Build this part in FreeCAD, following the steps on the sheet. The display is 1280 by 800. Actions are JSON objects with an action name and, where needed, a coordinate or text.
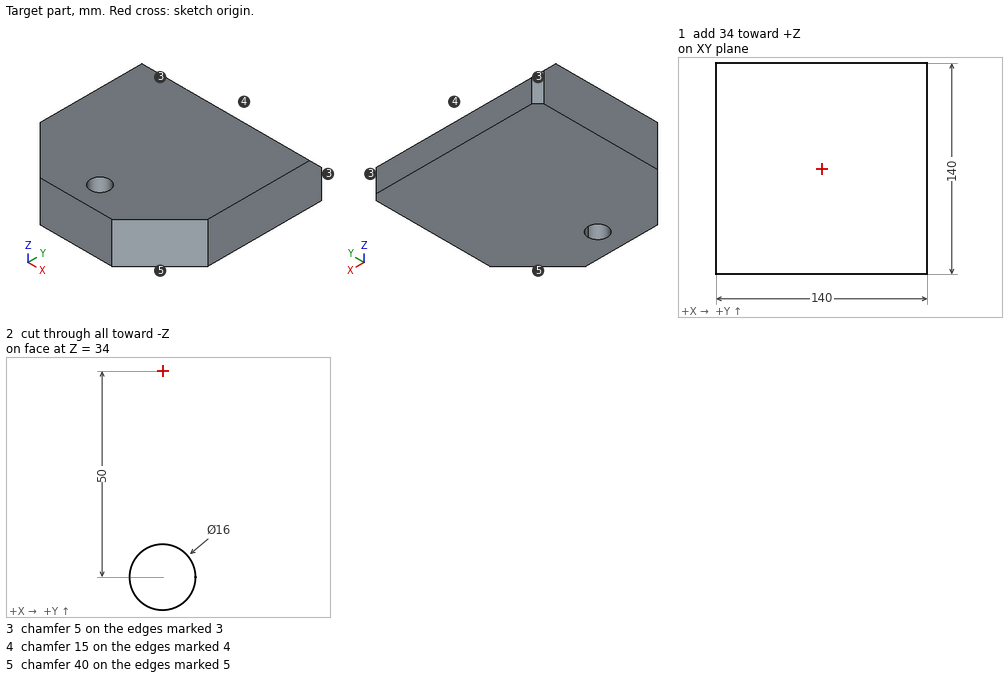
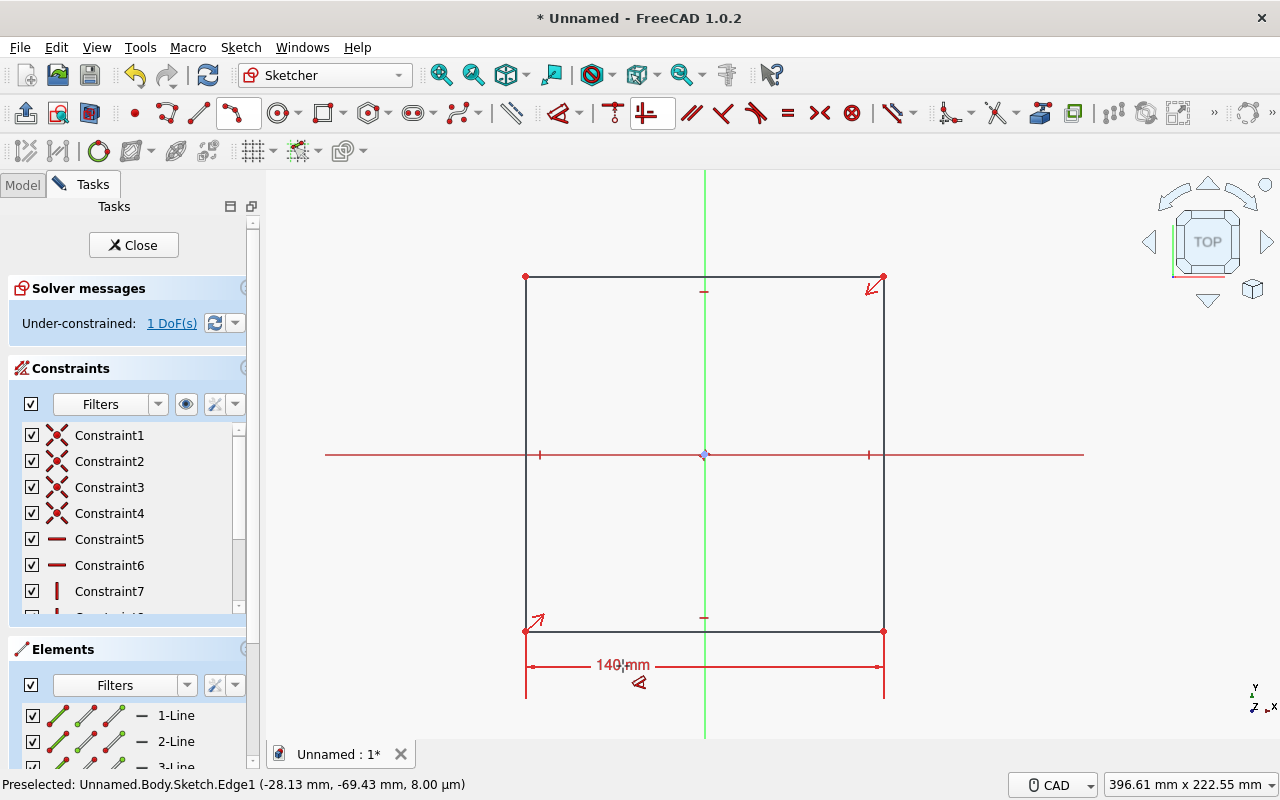
{"action": "left_click", "coordinate": [884, 526]}
{"action": "left_click", "coordinate": [918, 373]}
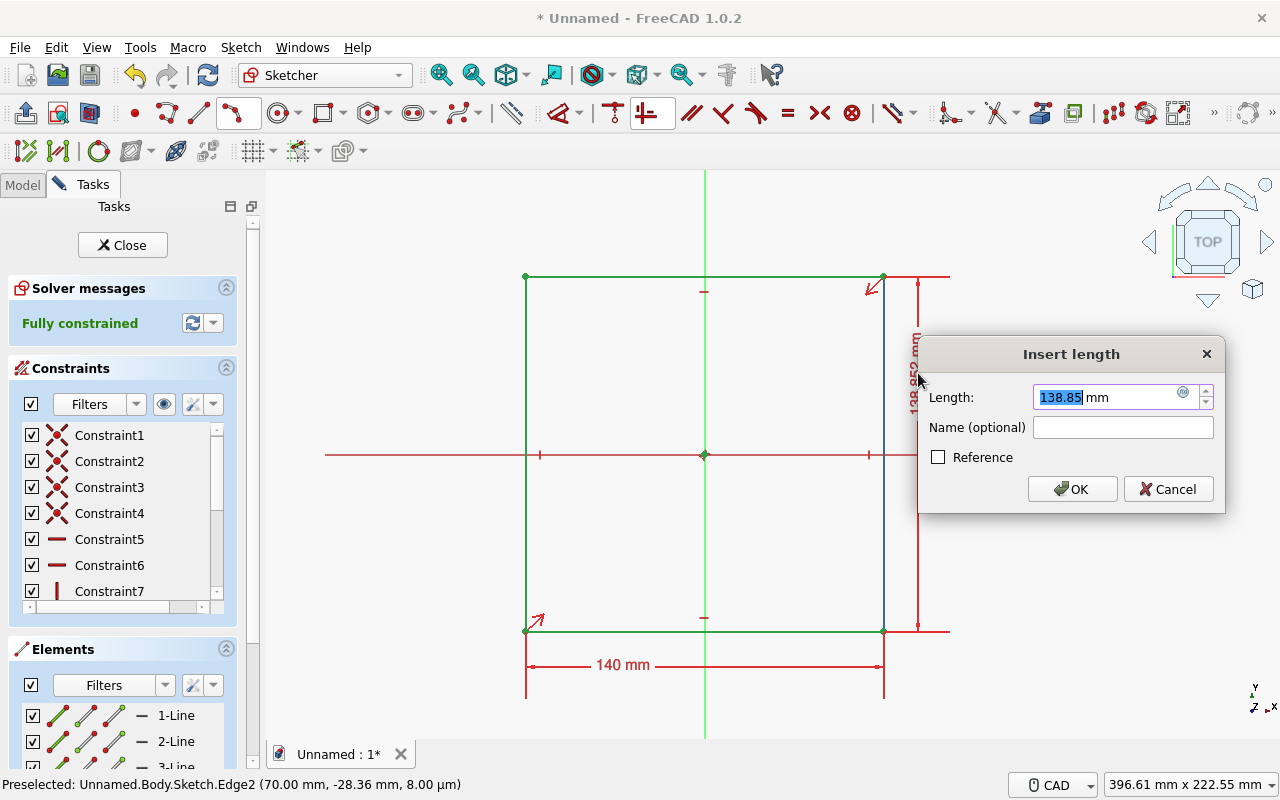
{"action": "type", "text": "140"}
{"action": "key", "text": "Return"}
{"action": "key", "text": "Escape"}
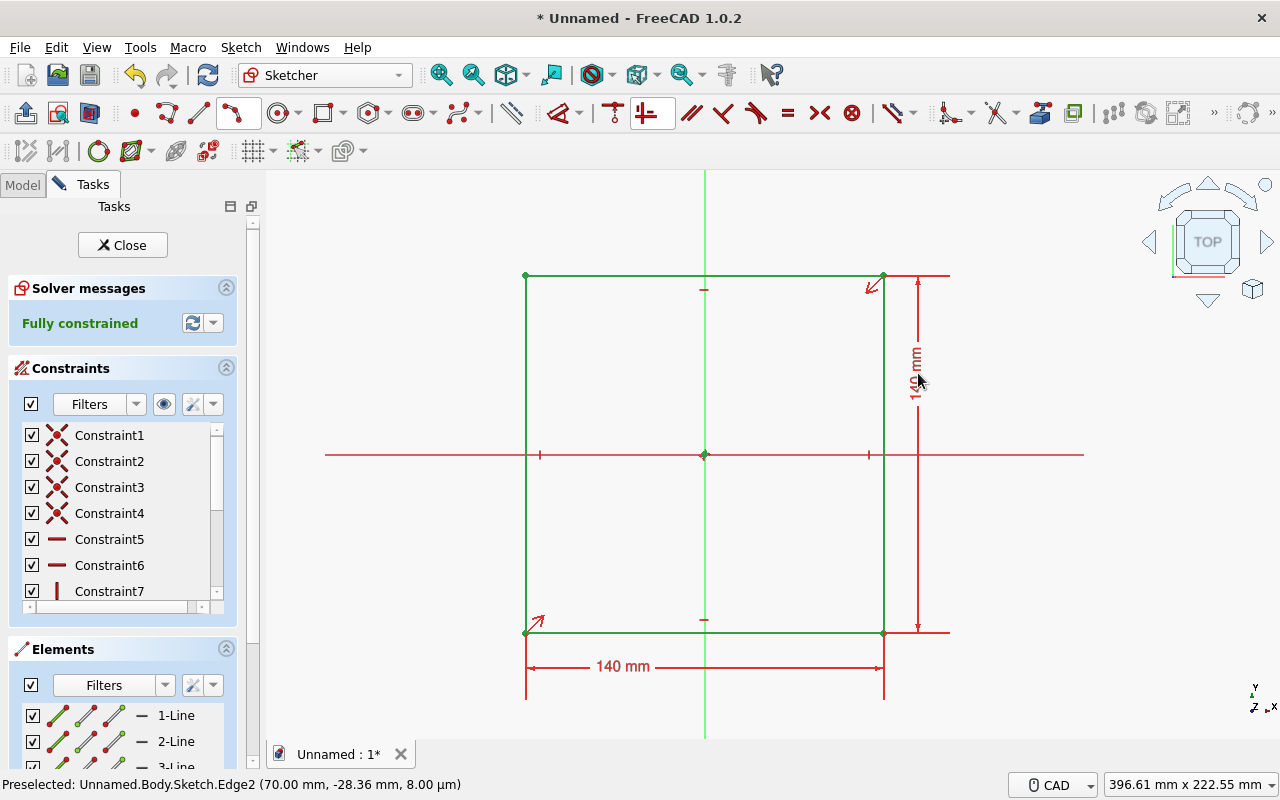
{"action": "left_click", "coordinate": [123, 245]}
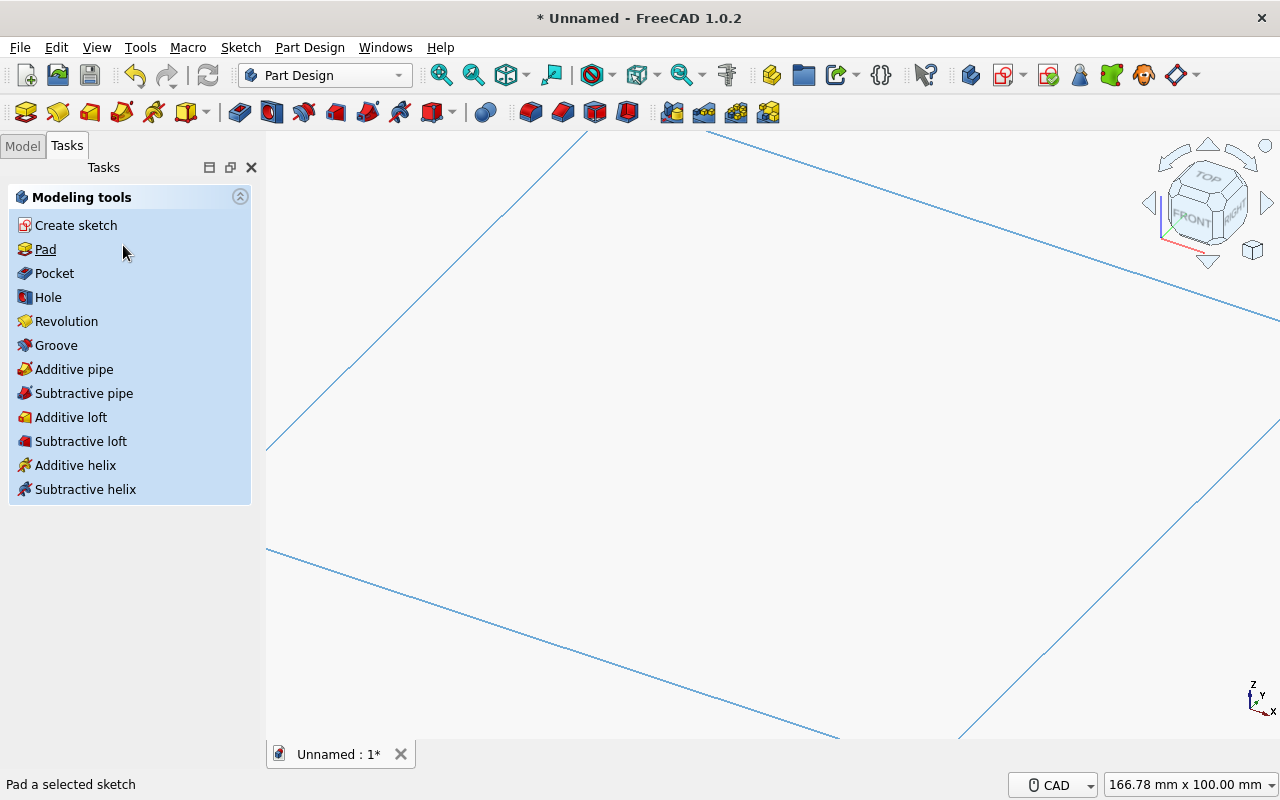
{"action": "left_click", "coordinate": [26, 112]}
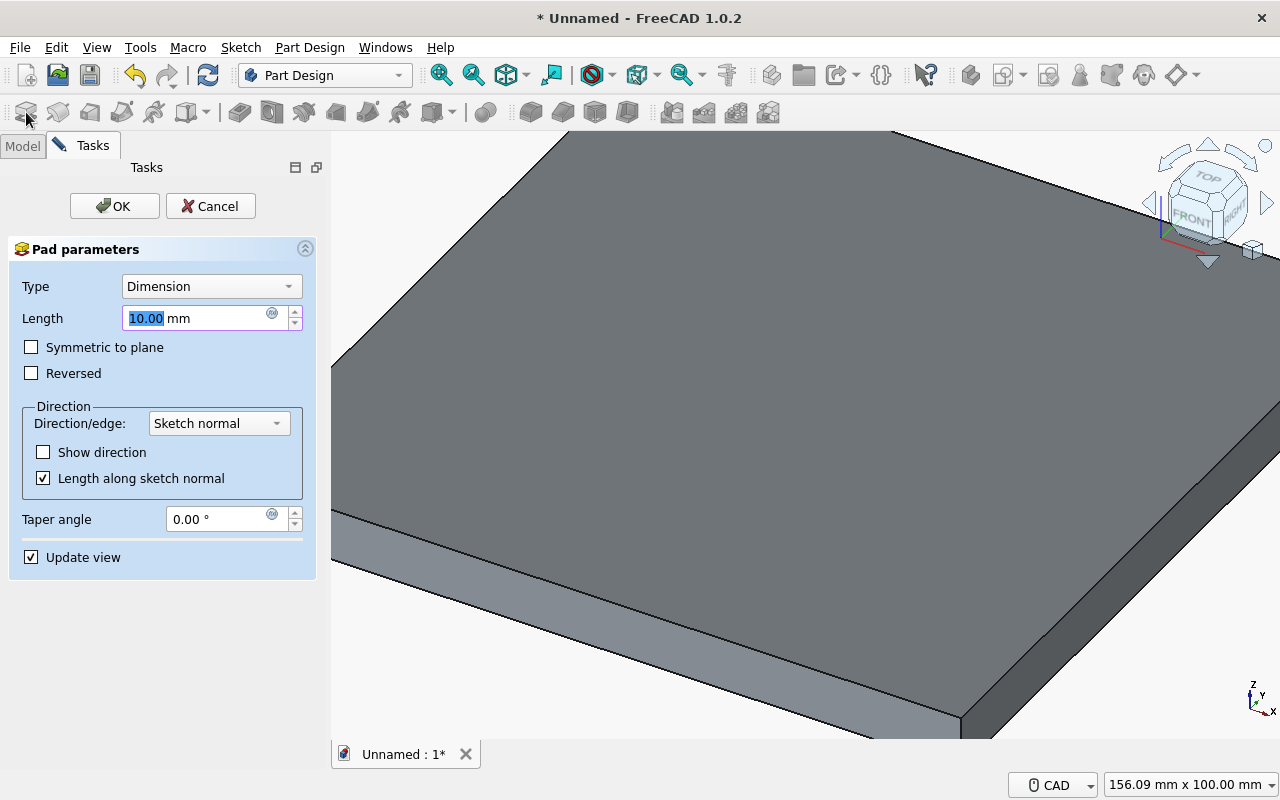
{"action": "type", "text": "34"}
{"action": "key", "text": "Tab"}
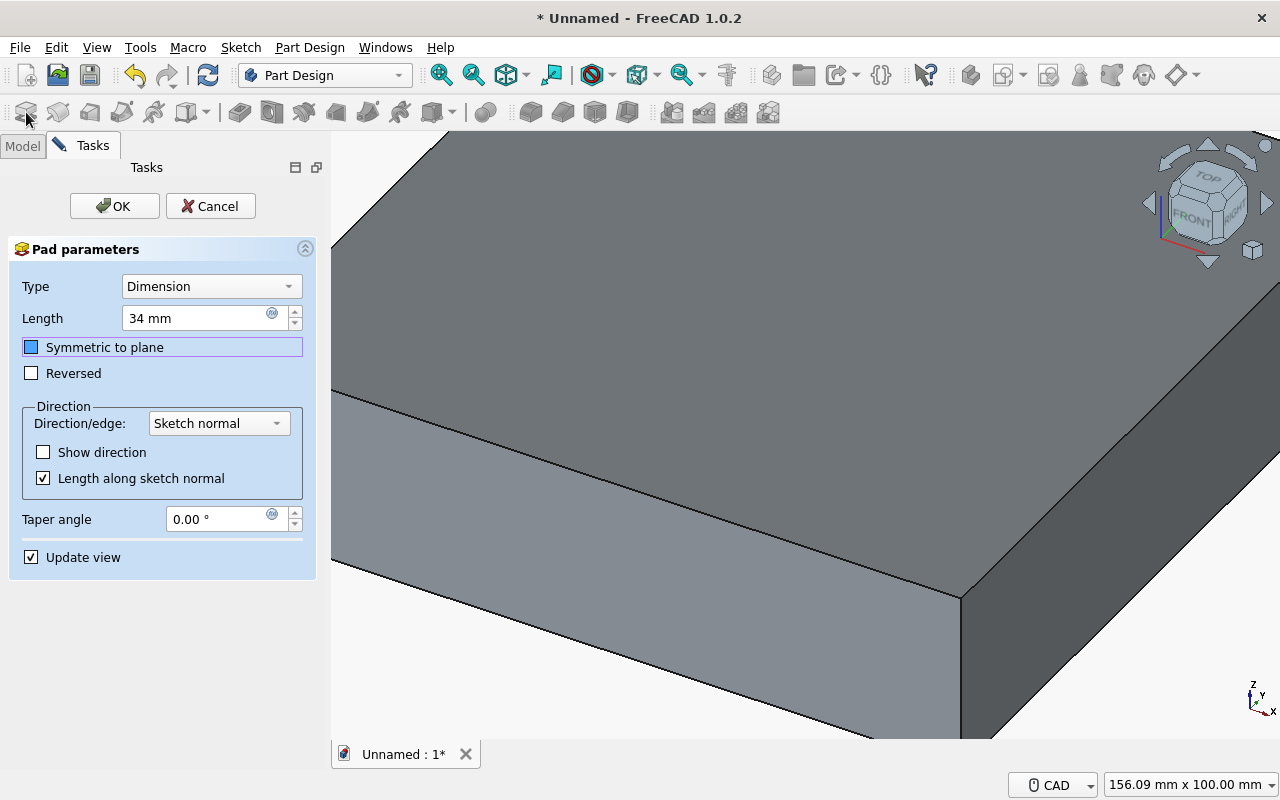
{"action": "left_click", "coordinate": [115, 206]}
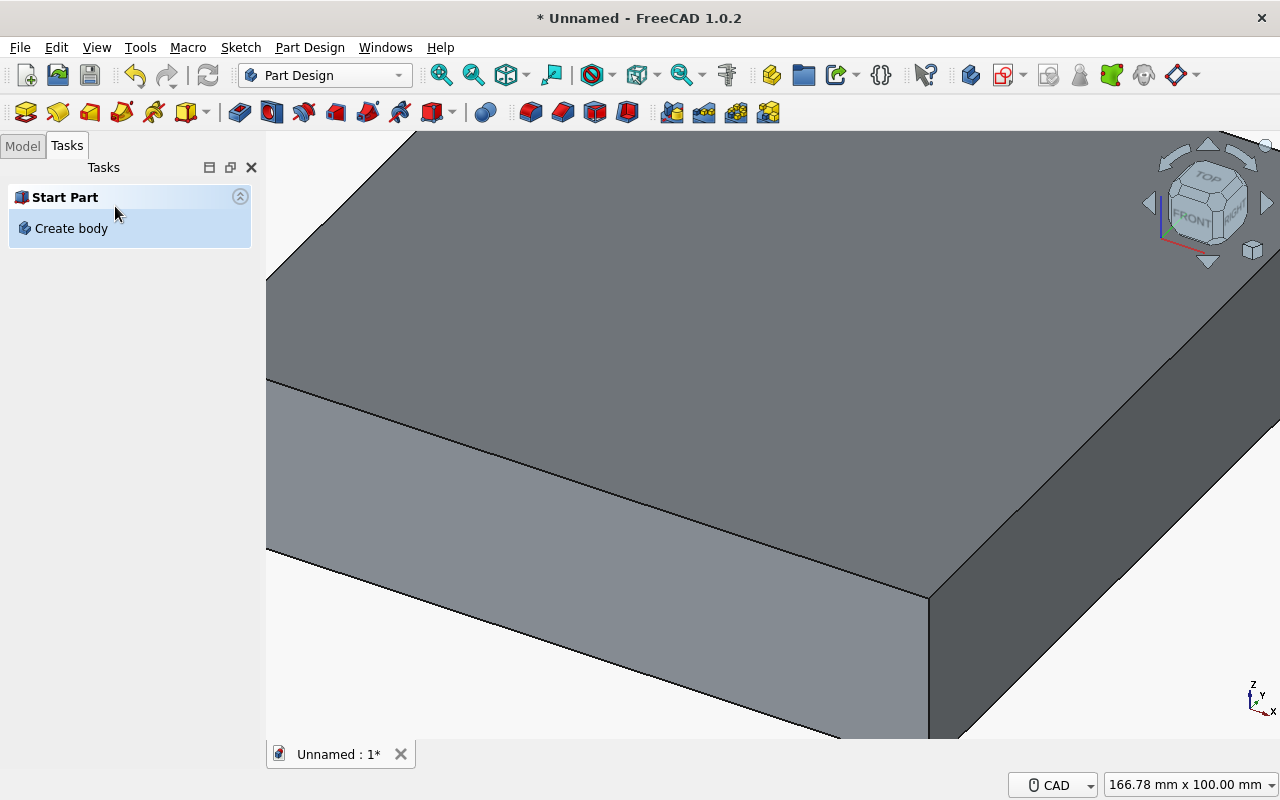
{"action": "left_click", "coordinate": [442, 76]}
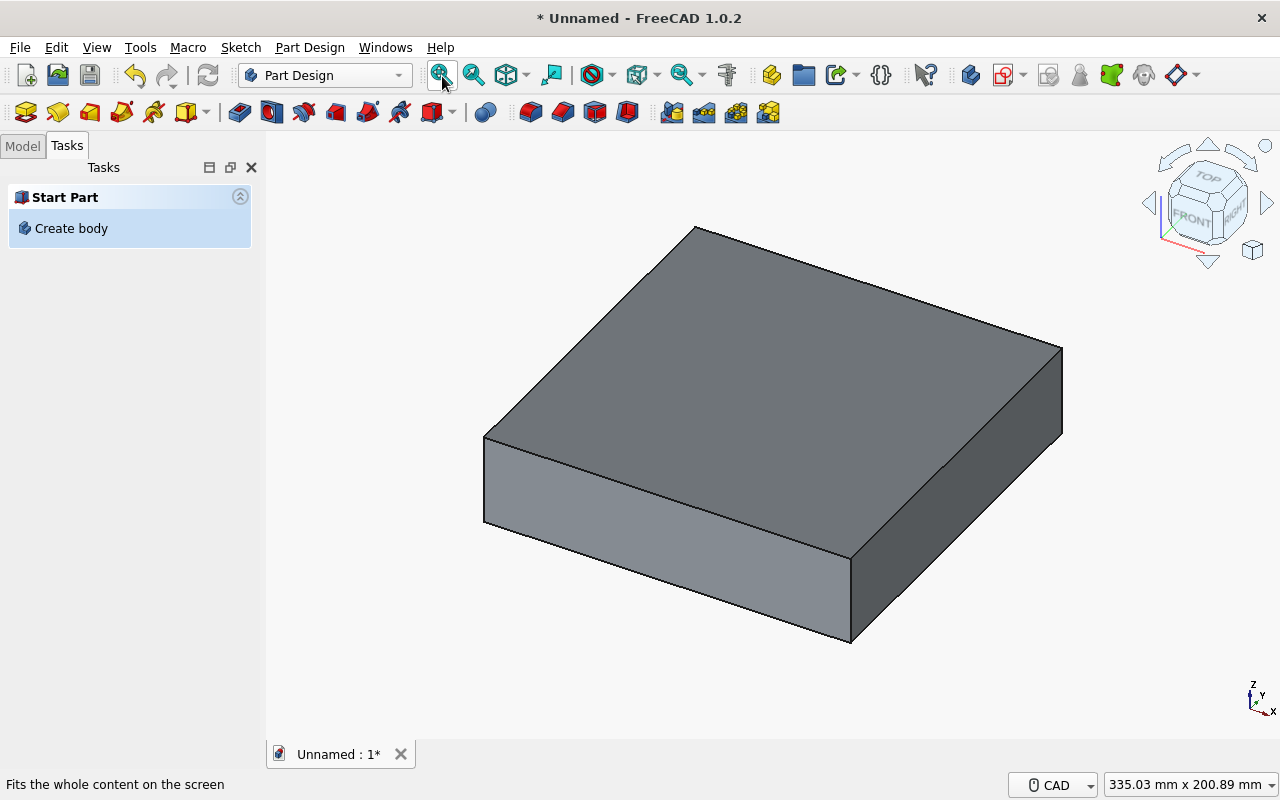
{"action": "left_click", "coordinate": [773, 392]}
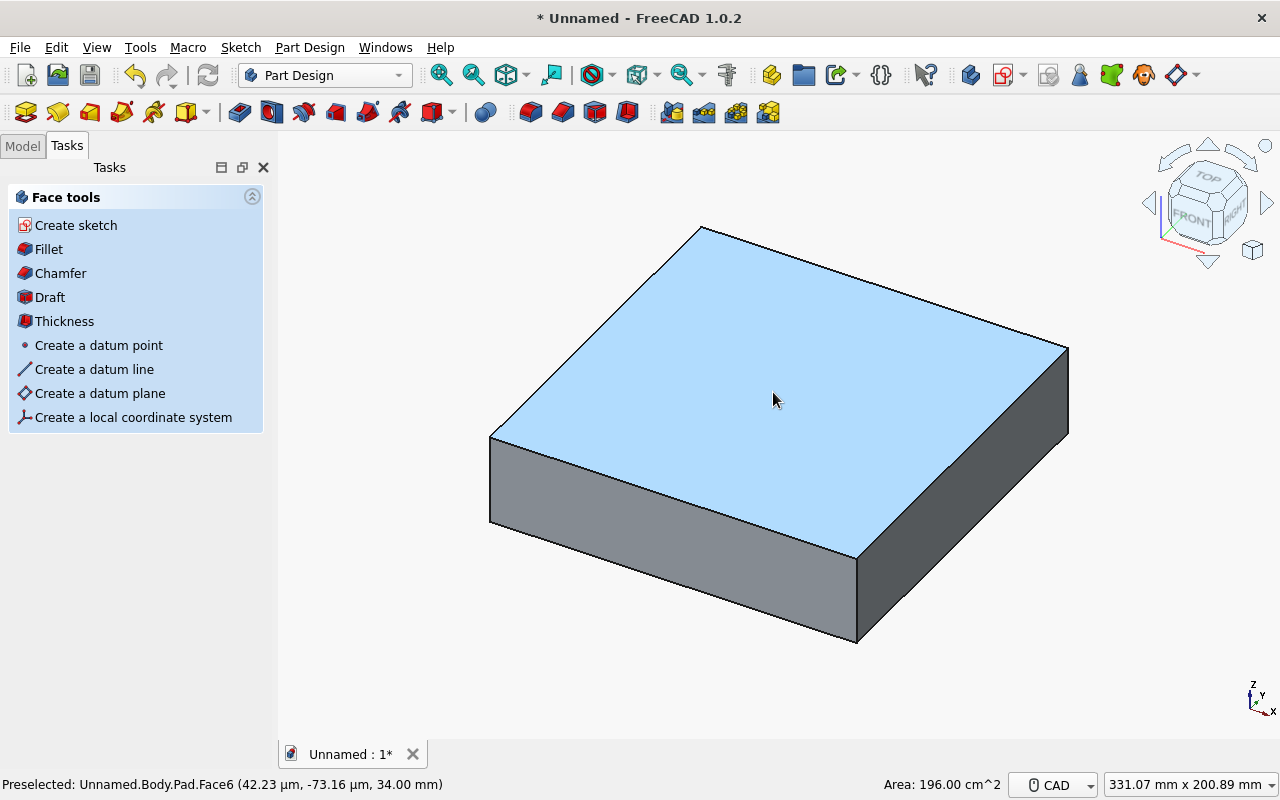
{"action": "left_click", "coordinate": [1004, 76]}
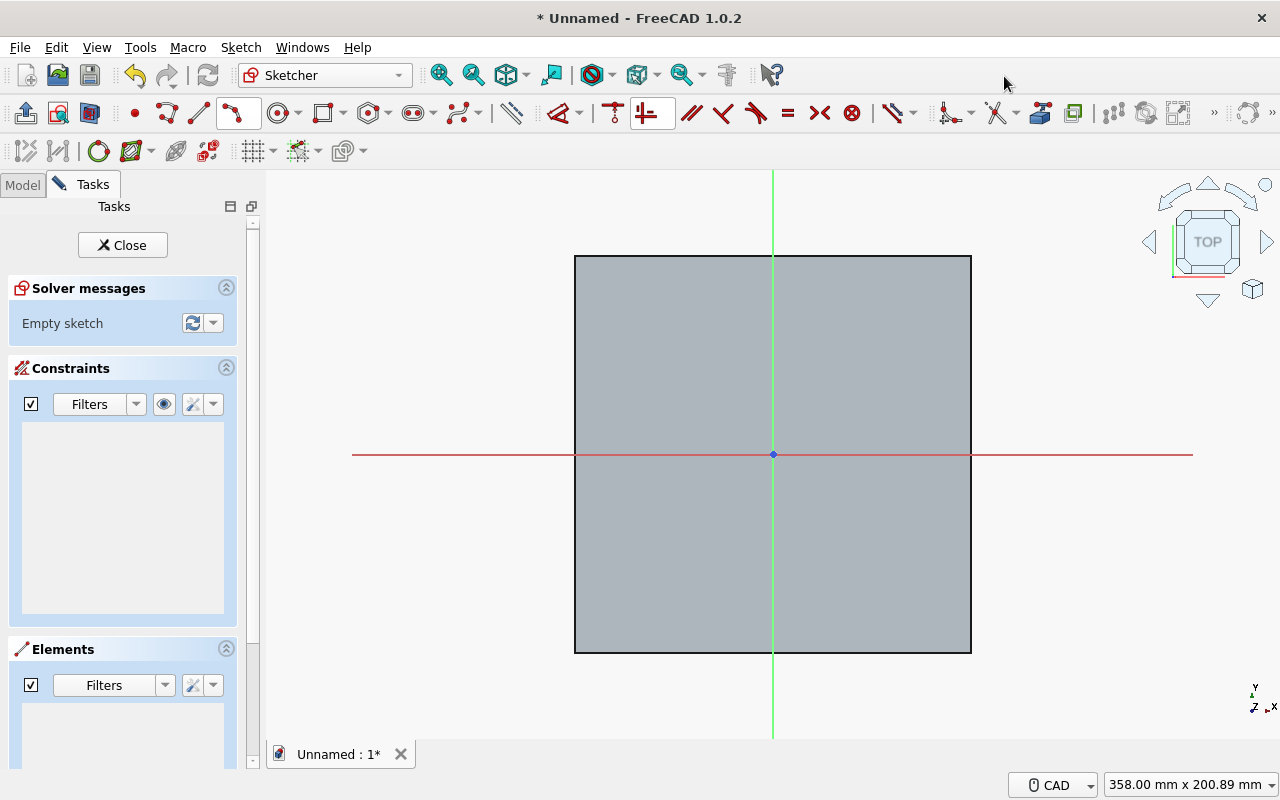
{"action": "scroll", "coordinate": [784, 618], "scroll_direction": "up", "scroll_amount": 10}